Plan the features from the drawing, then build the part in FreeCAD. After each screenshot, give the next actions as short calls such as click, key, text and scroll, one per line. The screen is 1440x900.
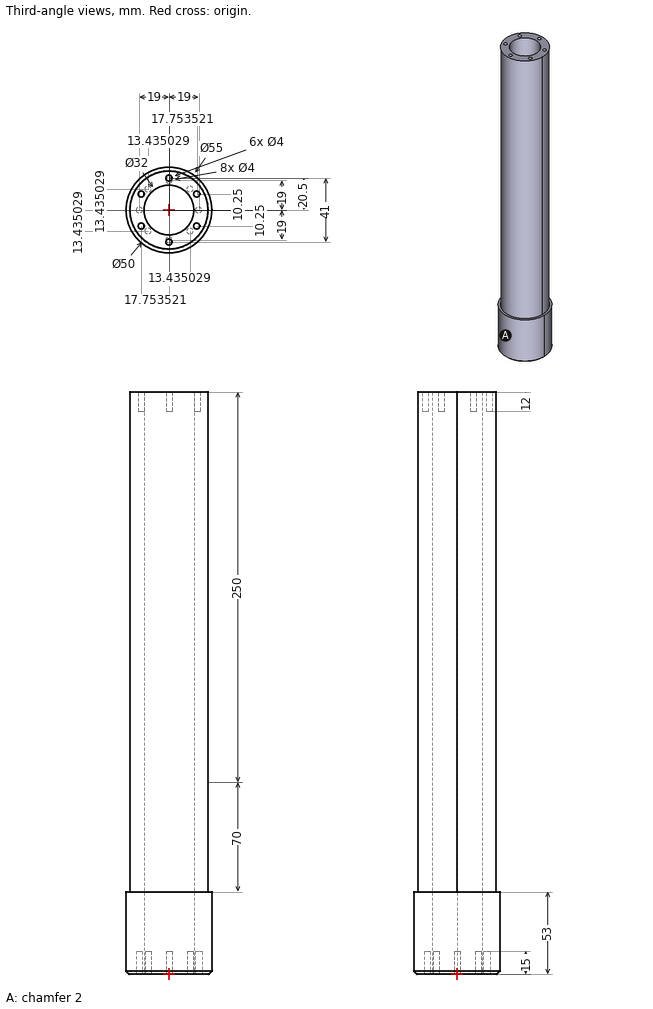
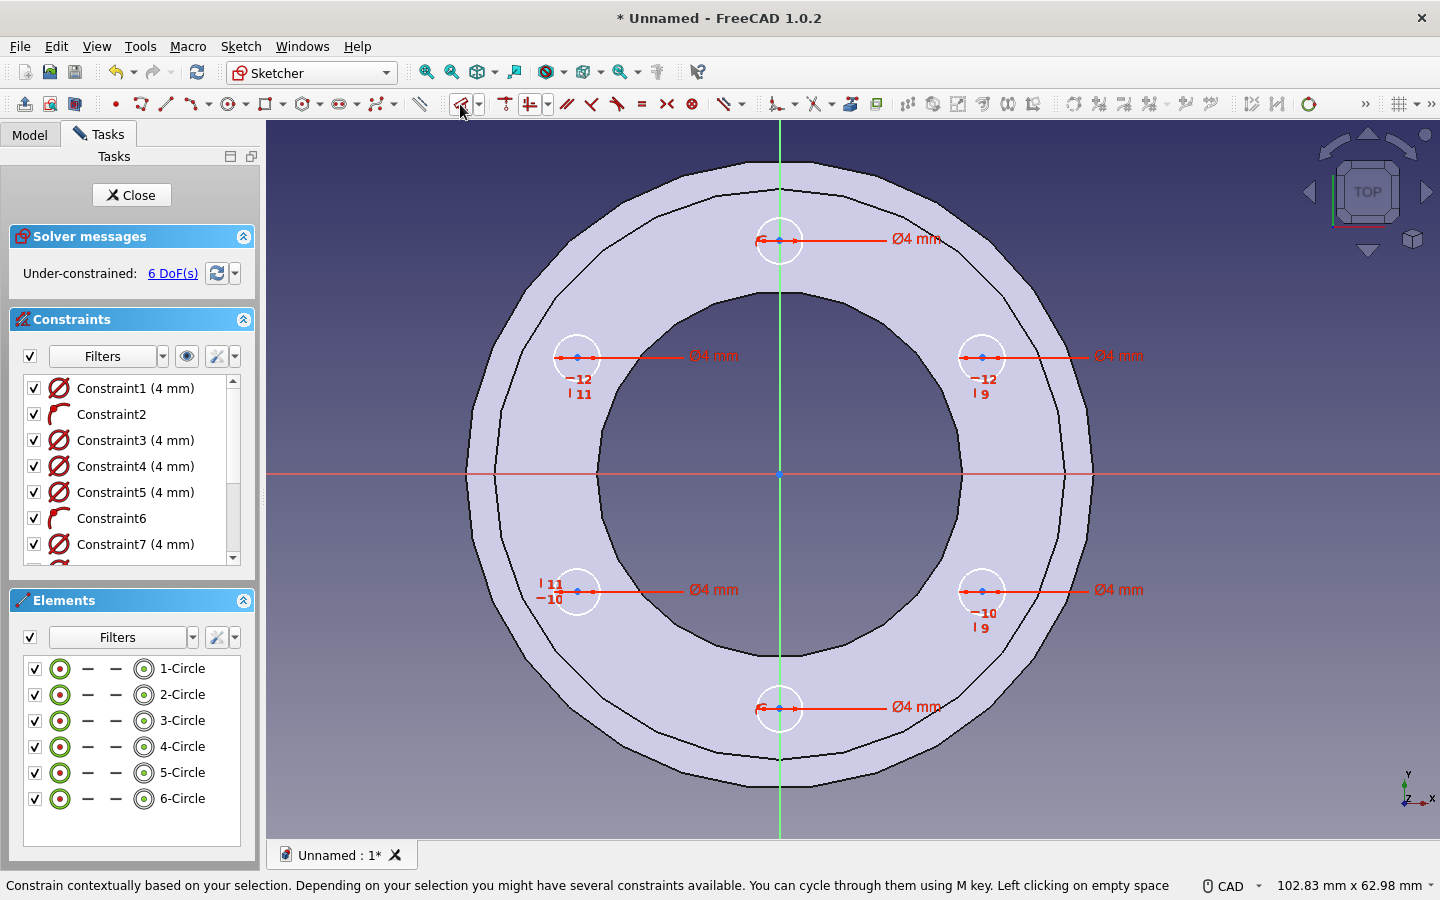
click(780, 241)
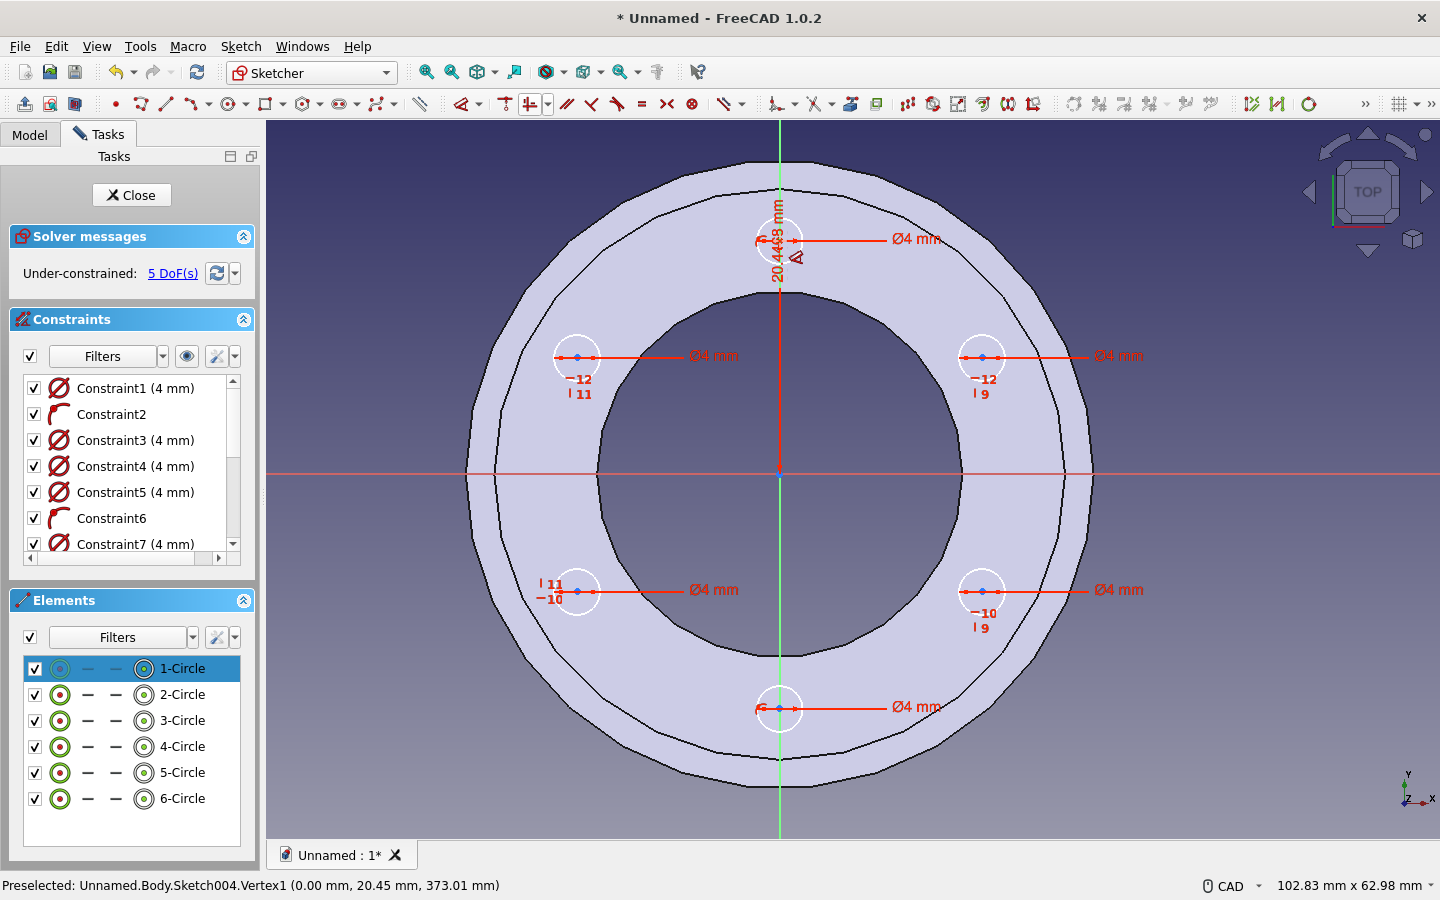
click(780, 709)
click(814, 367)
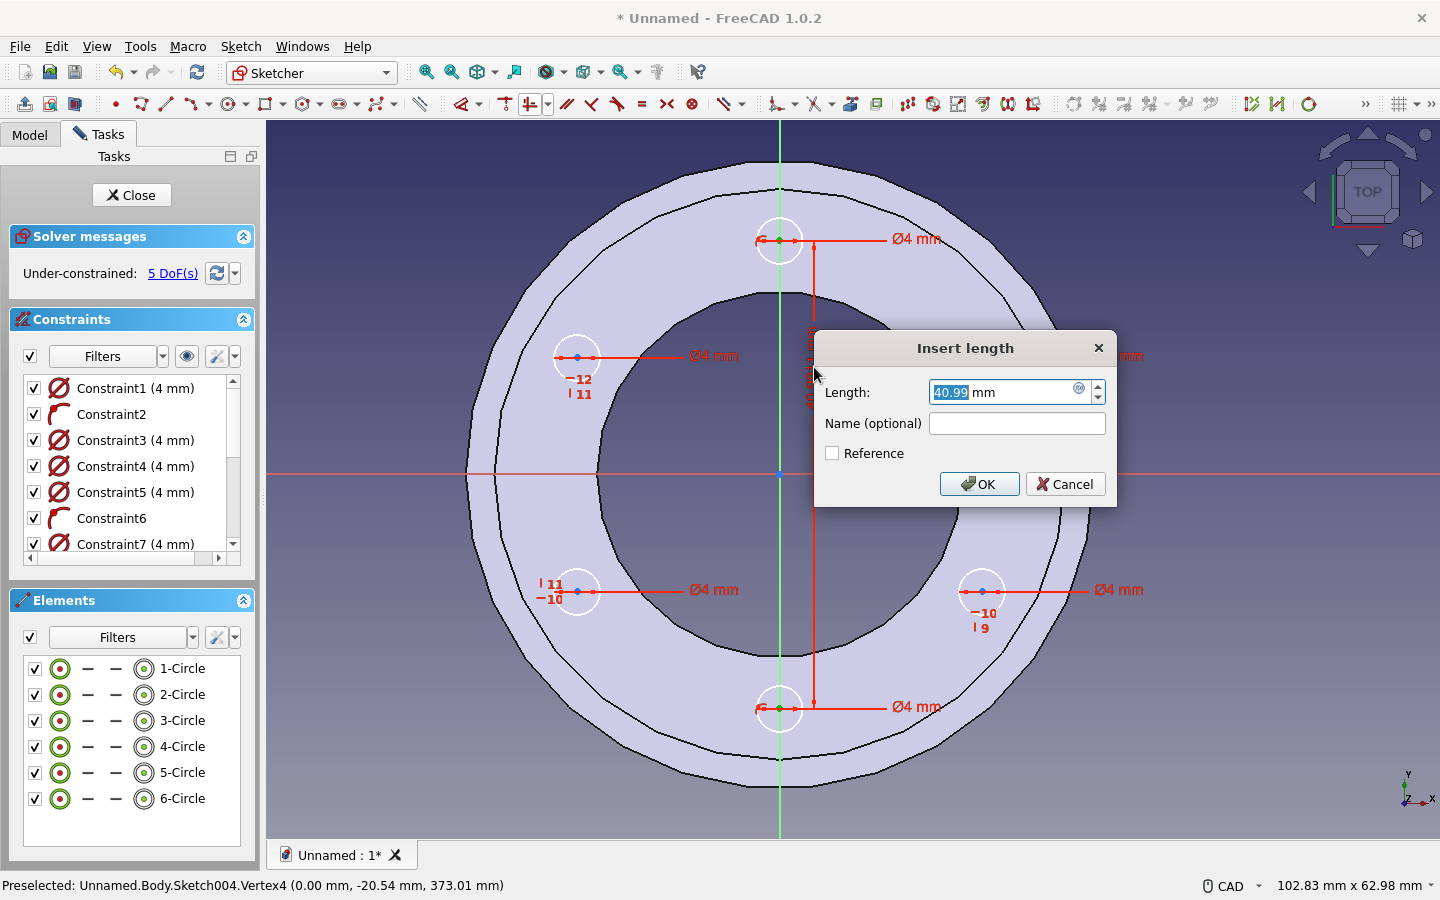
text(41)
key(Return)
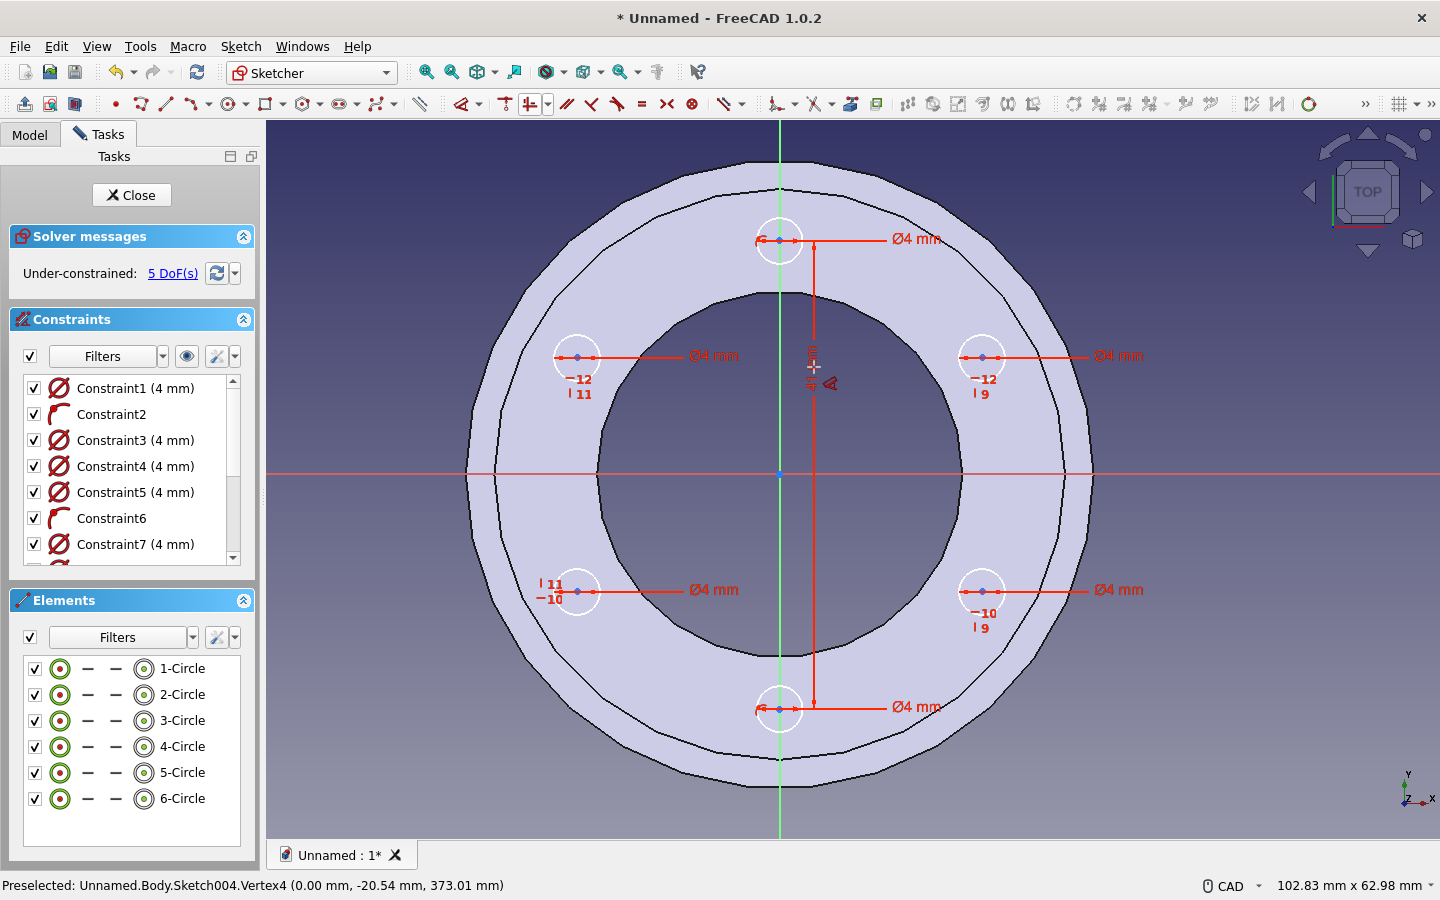
click(780, 241)
click(814, 304)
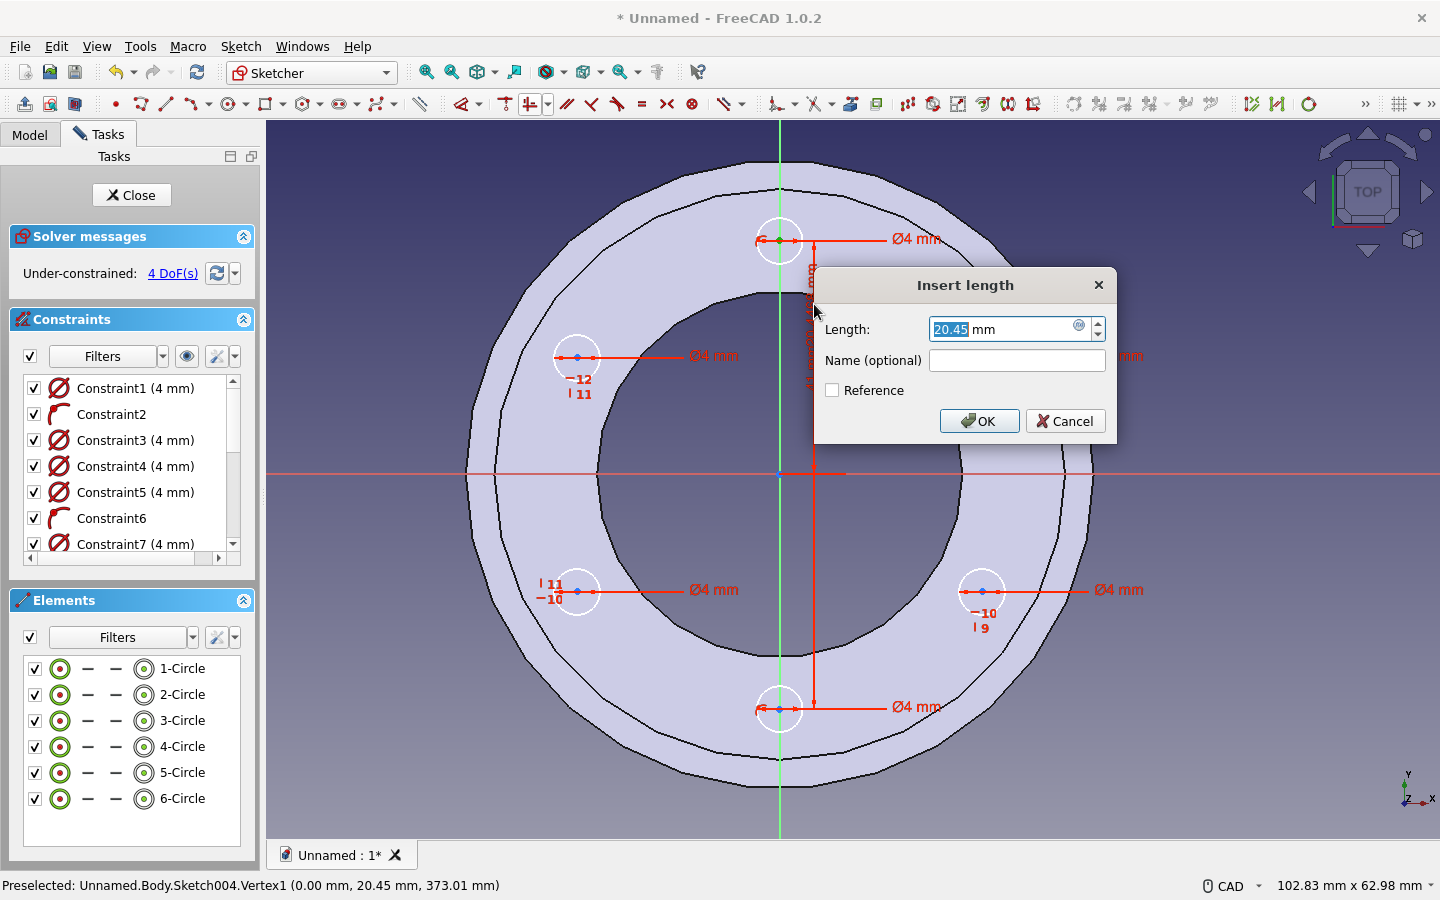
text(20.5)
key(Return)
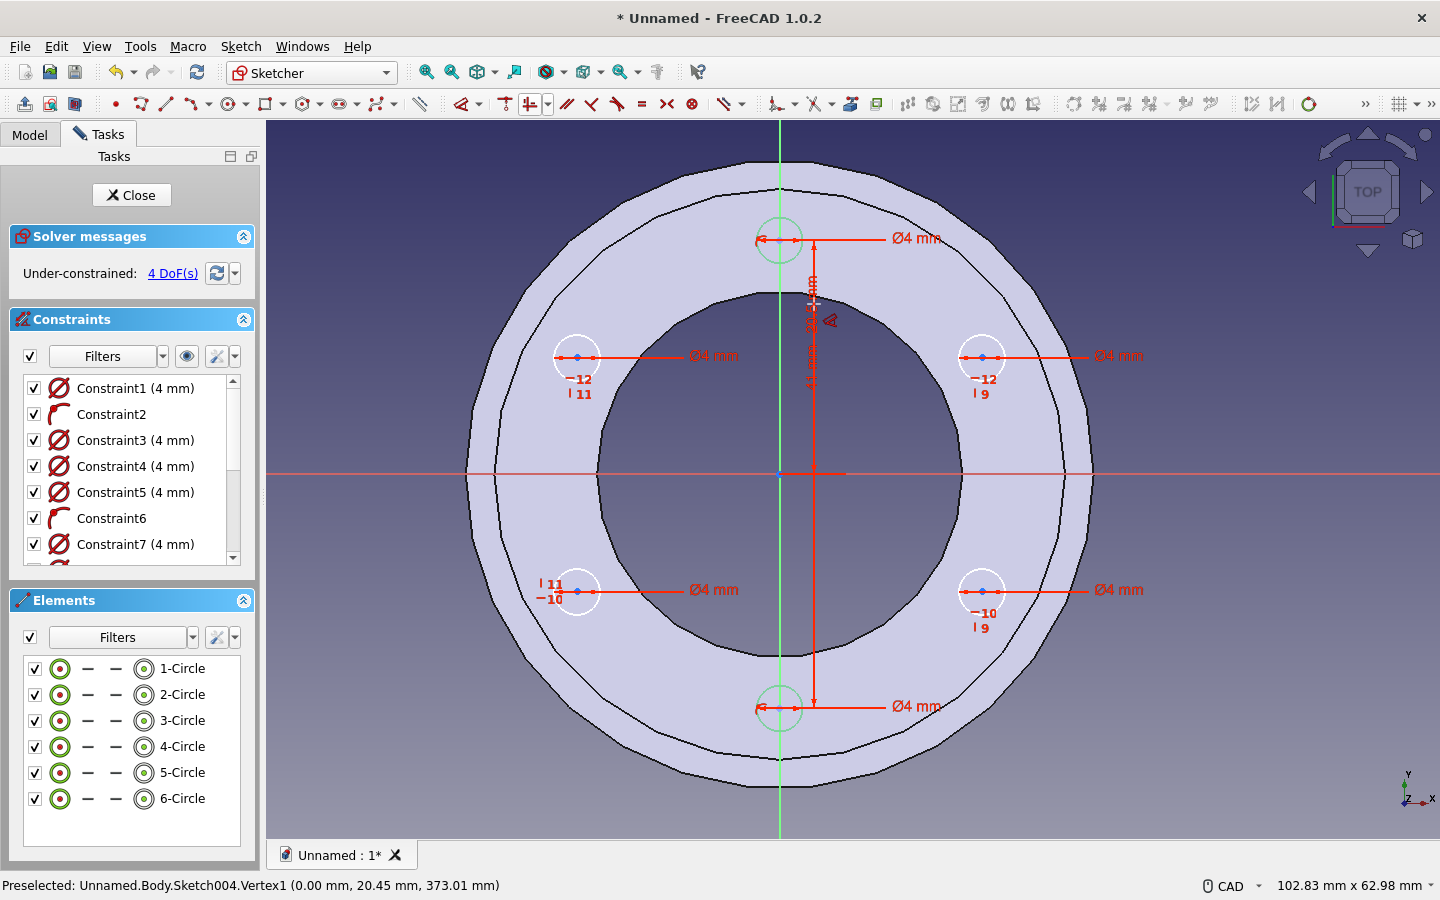
click(982, 358)
click(1016, 416)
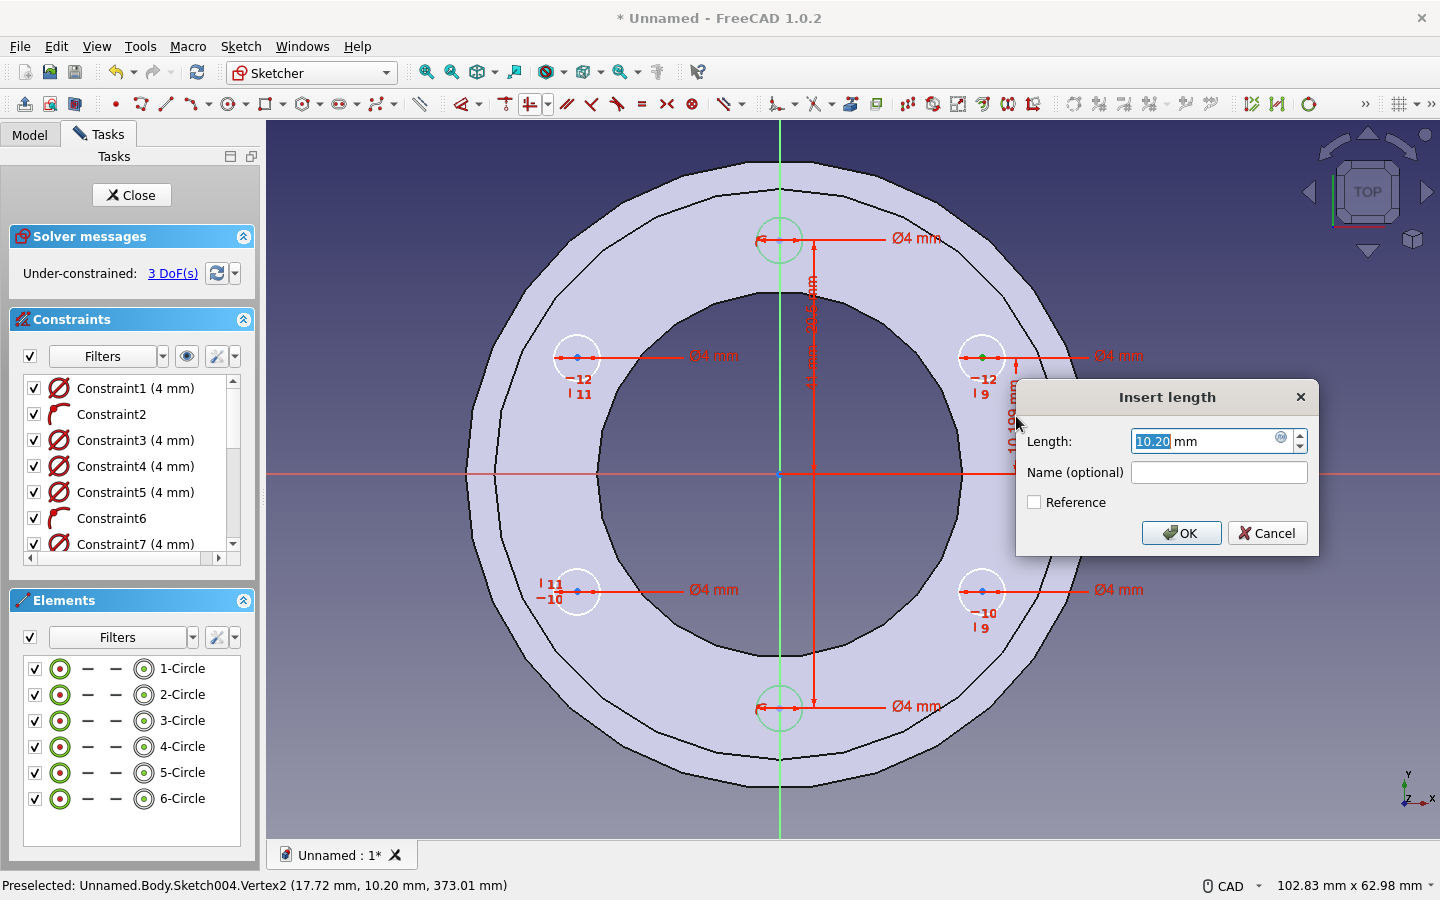
text(10.25)
key(Return)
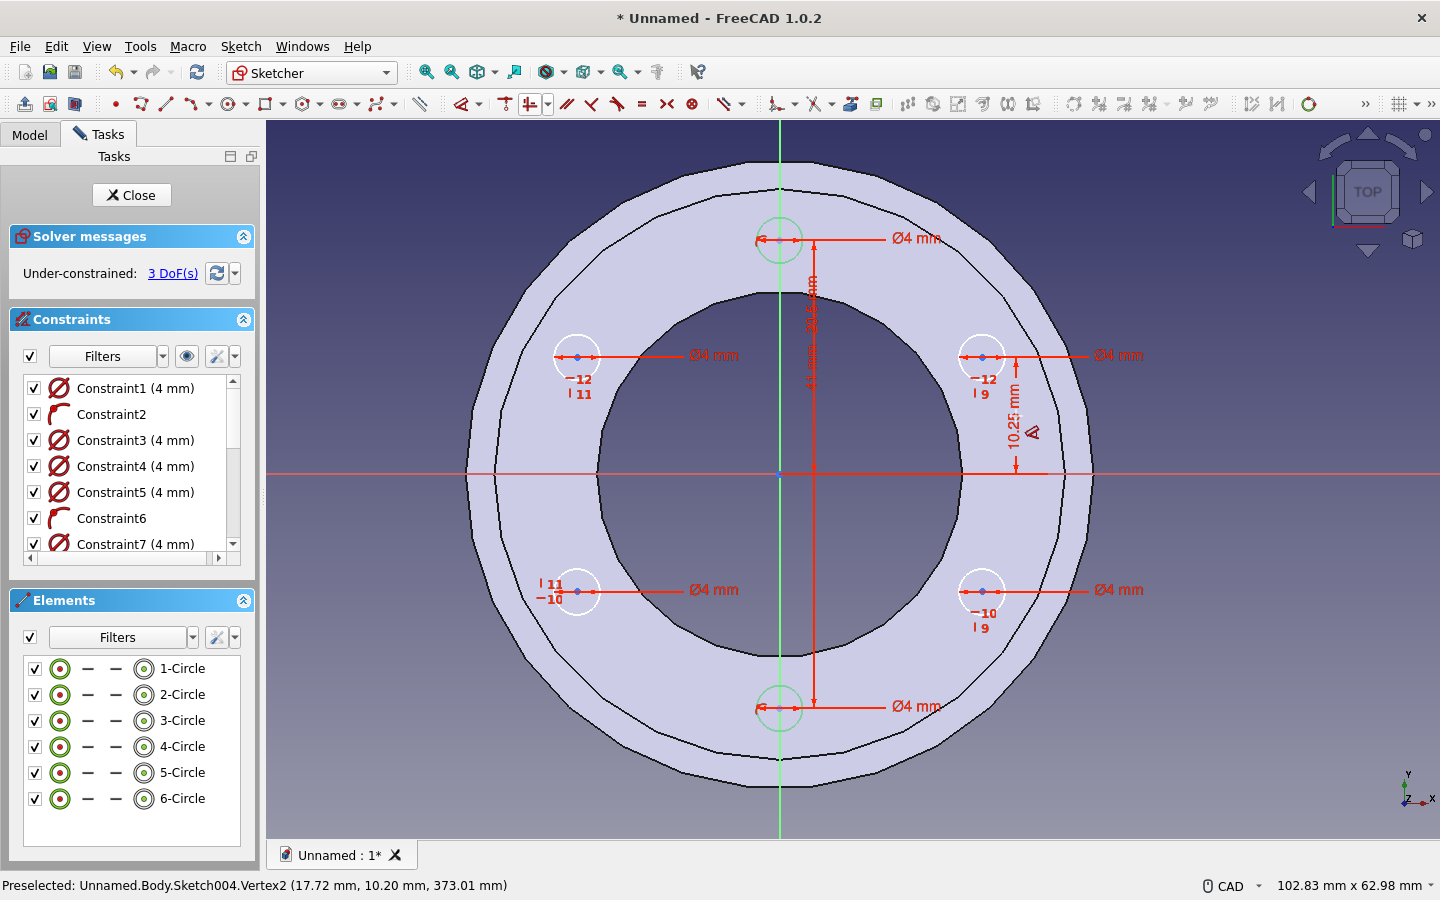
click(982, 592)
click(1016, 533)